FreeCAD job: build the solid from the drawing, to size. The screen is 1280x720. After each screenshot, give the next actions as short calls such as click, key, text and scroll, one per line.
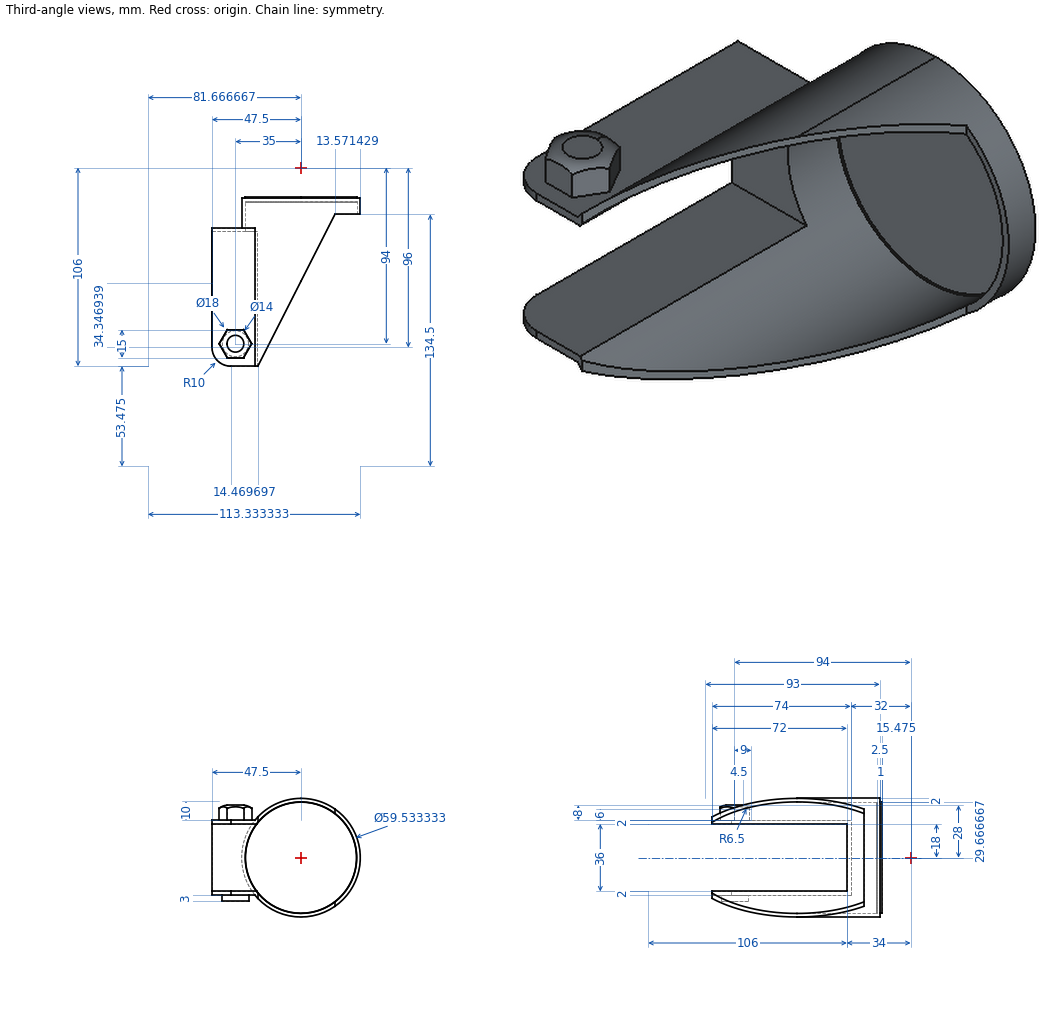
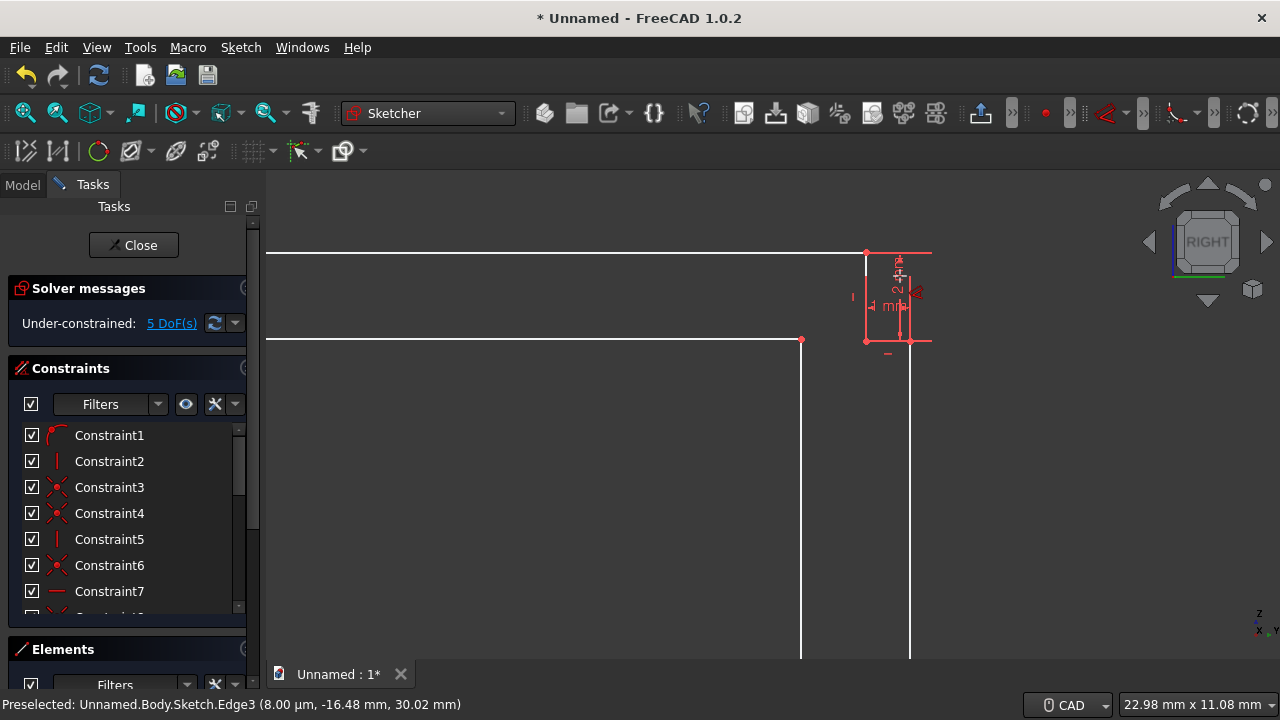
scroll(895, 348, down, 11)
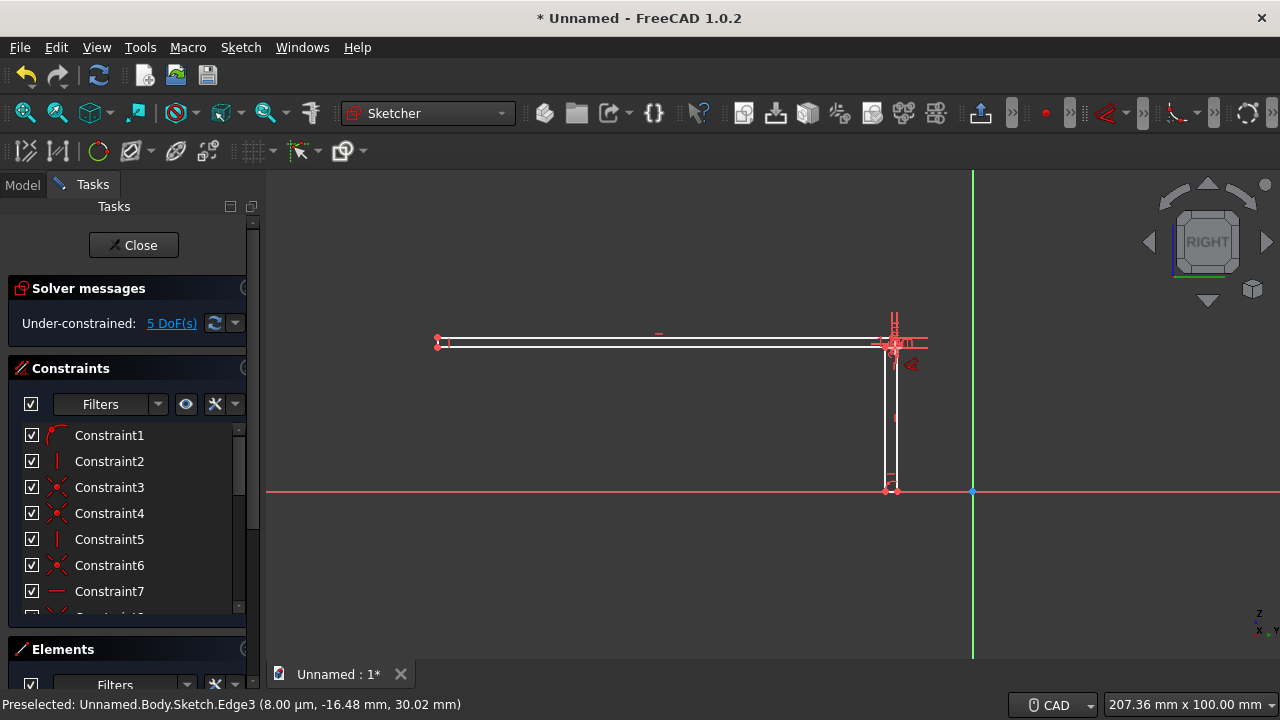
scroll(438, 341, up, 8)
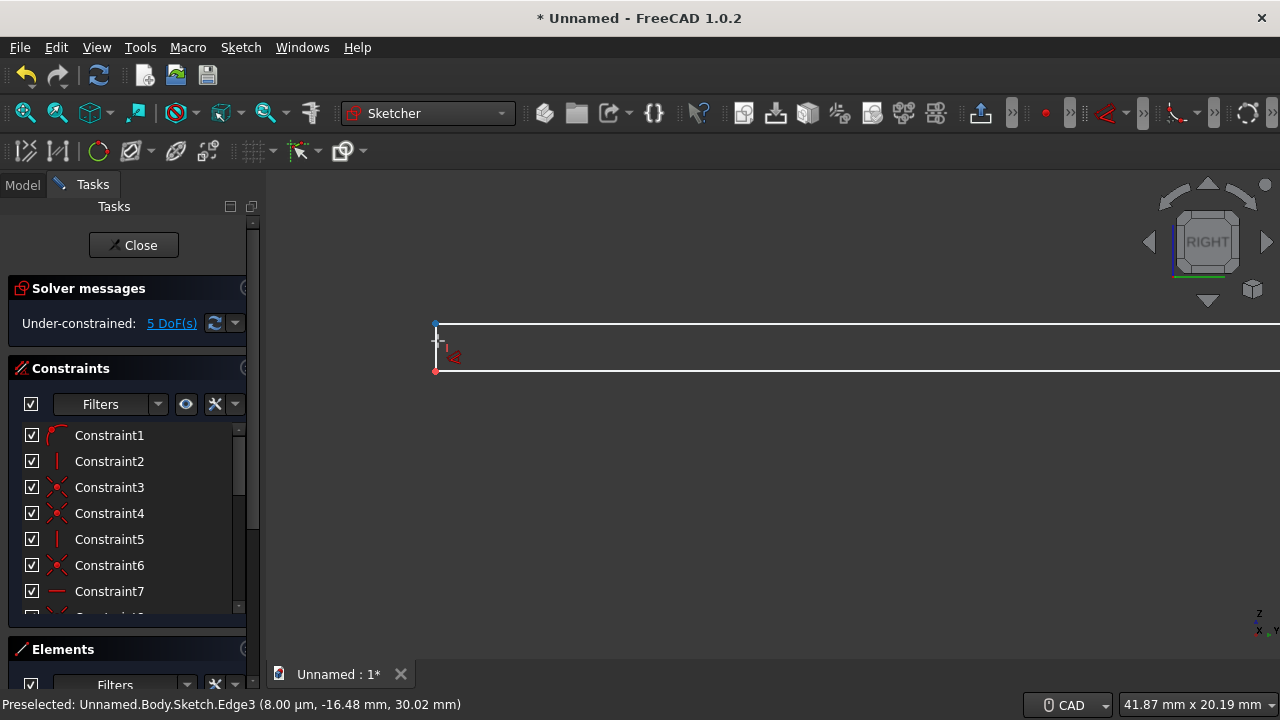
click(436, 338)
click(402, 347)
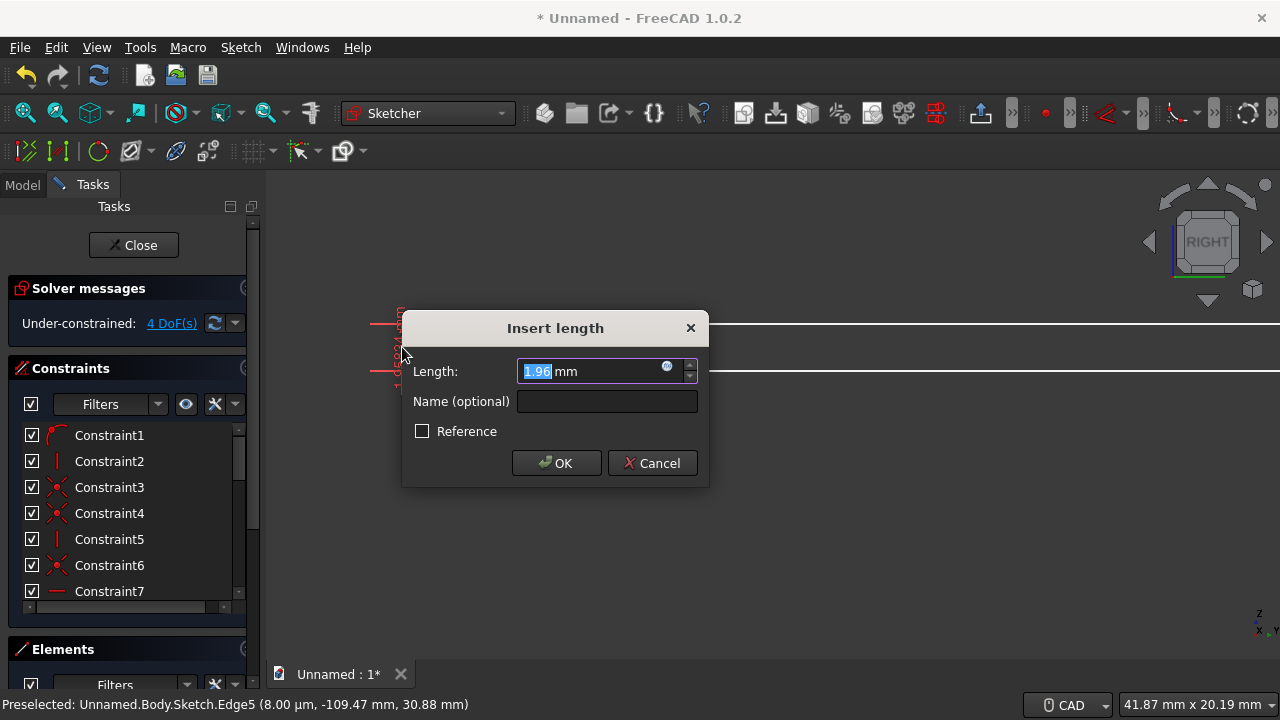
text(2)
key(Return)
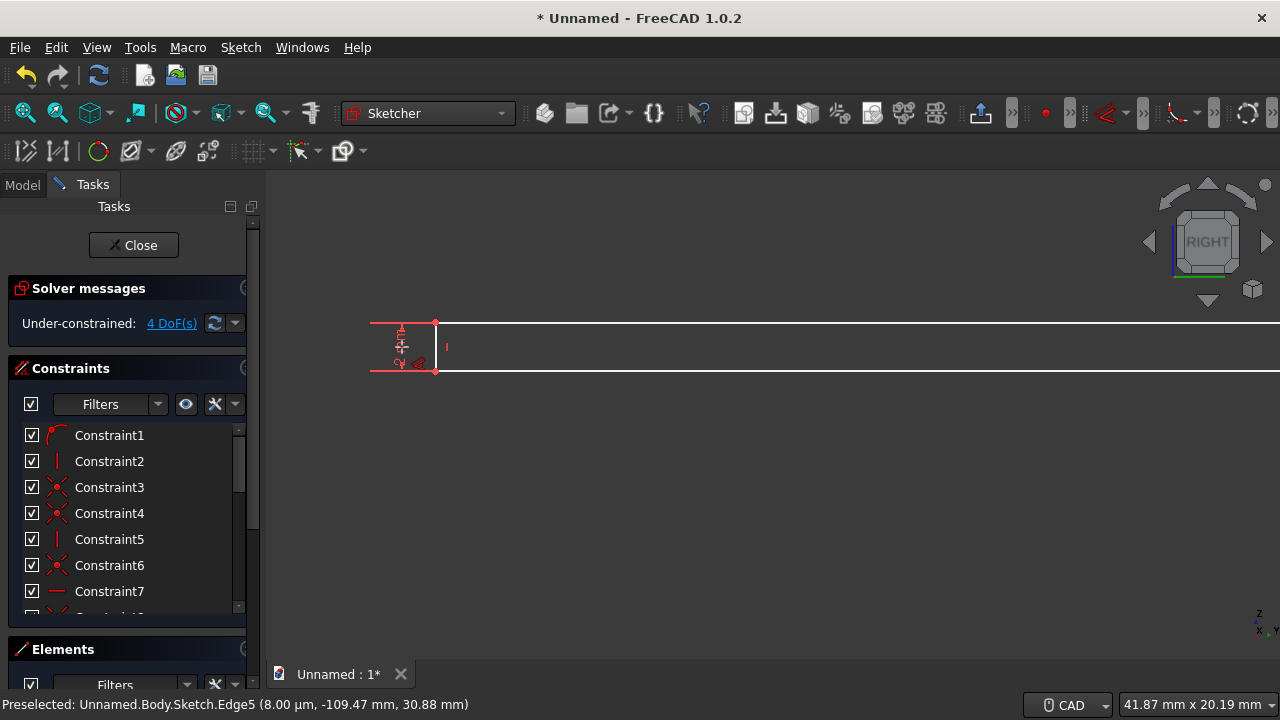
scroll(437, 341, down, 8)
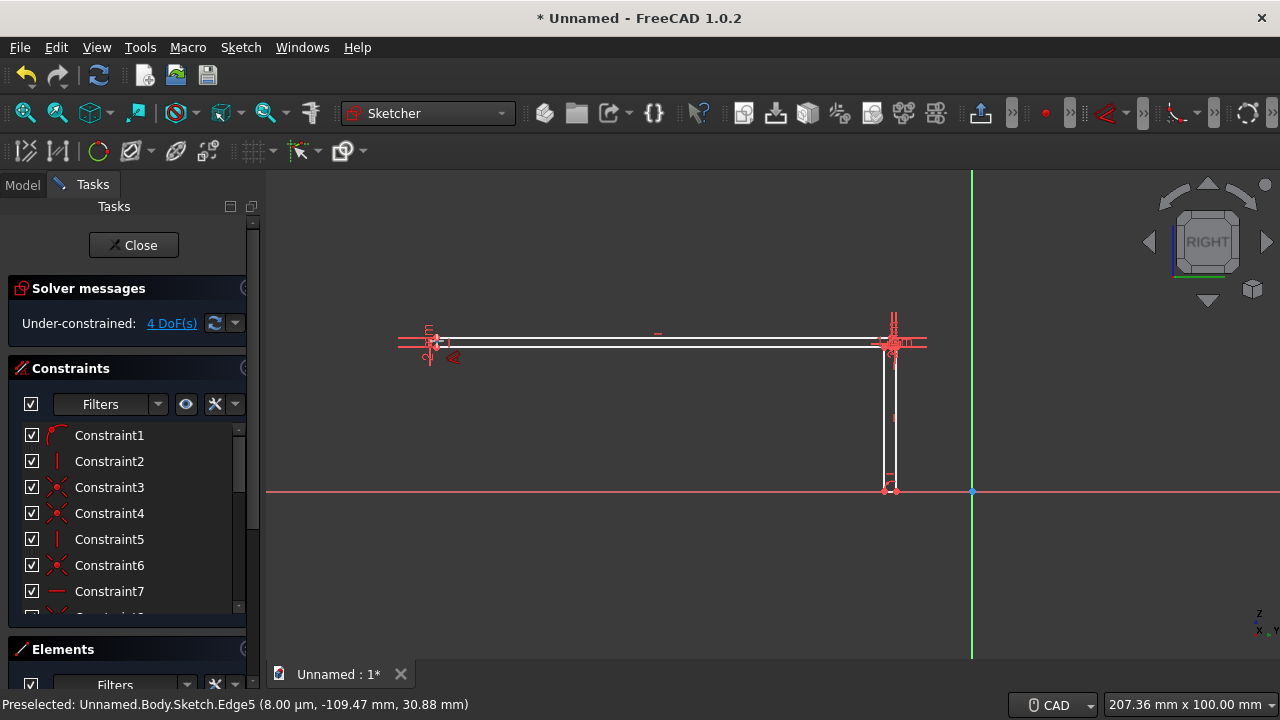
scroll(573, 338, up, 2)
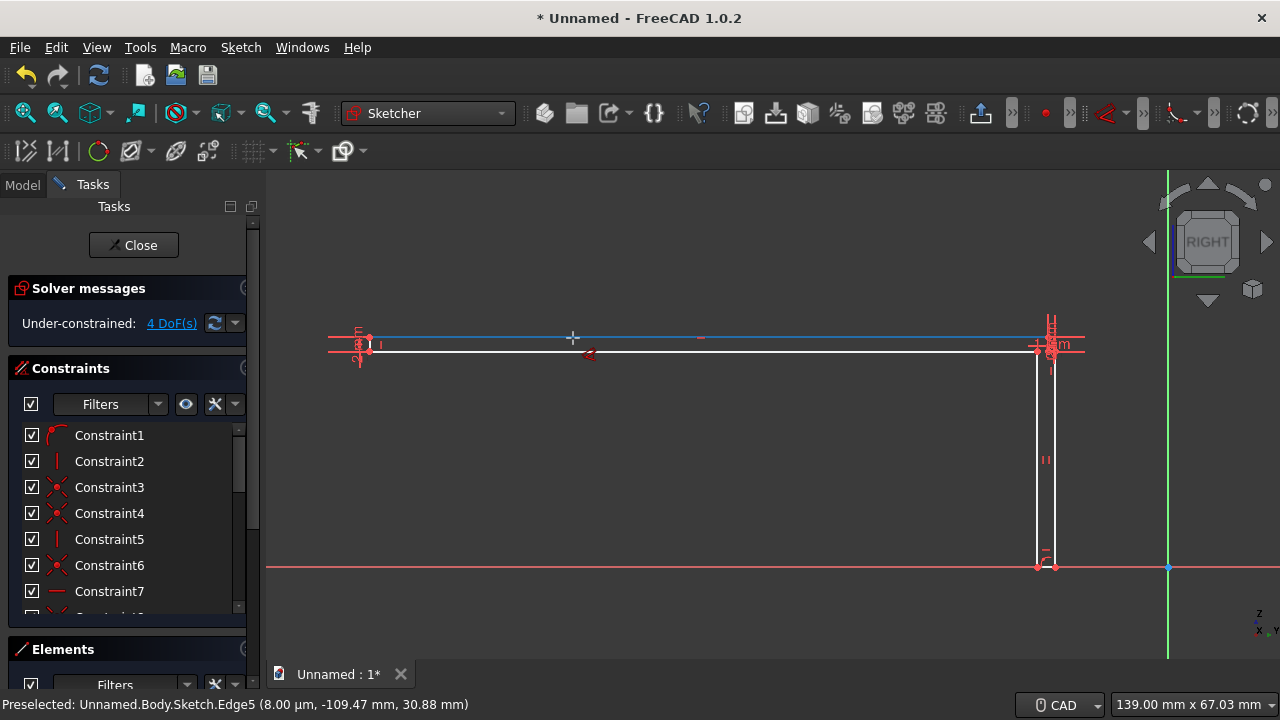
click(573, 337)
click(709, 303)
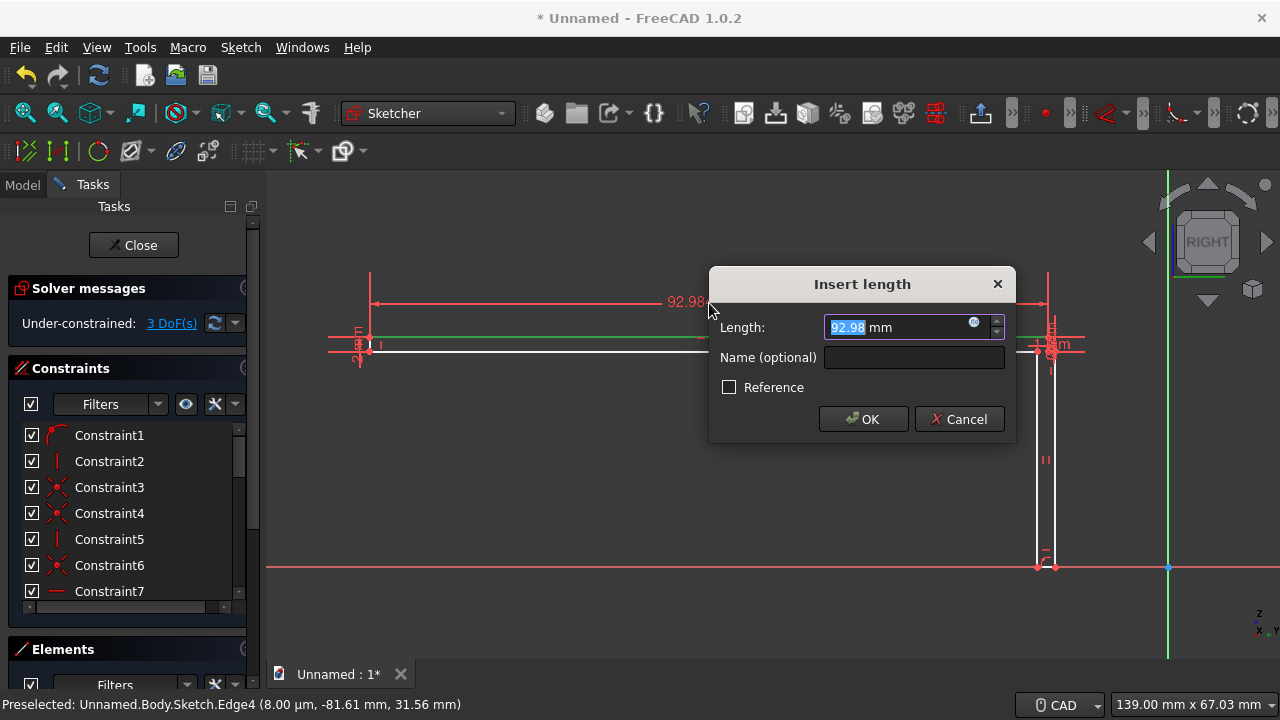
text(93)
key(Return)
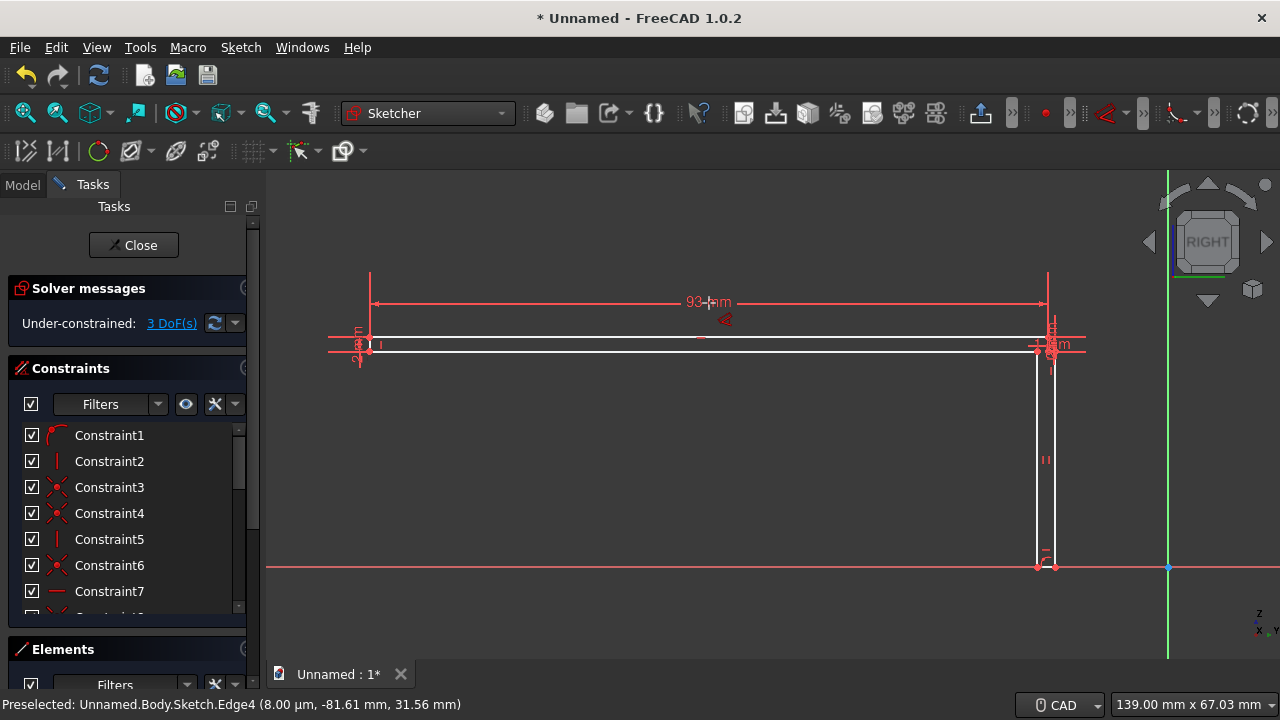
scroll(1046, 567, up, 4)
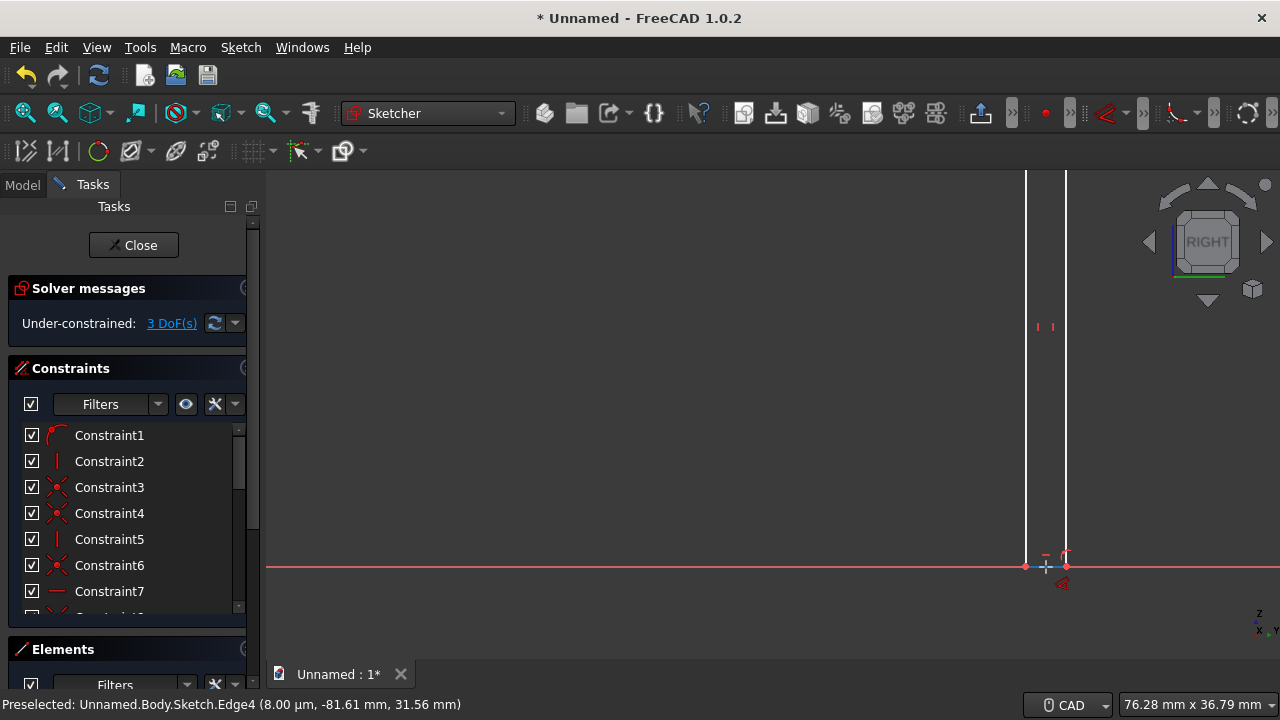
click(1046, 567)
click(1046, 601)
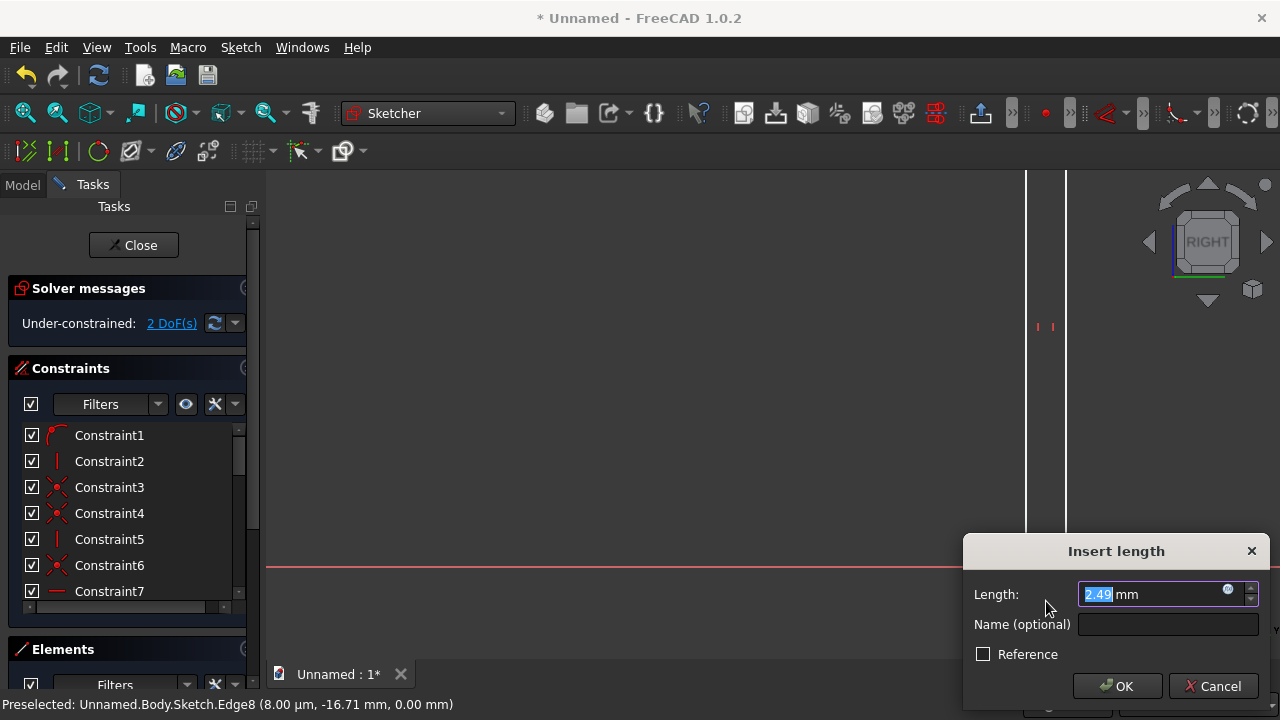
text(2.5)
key(Return)